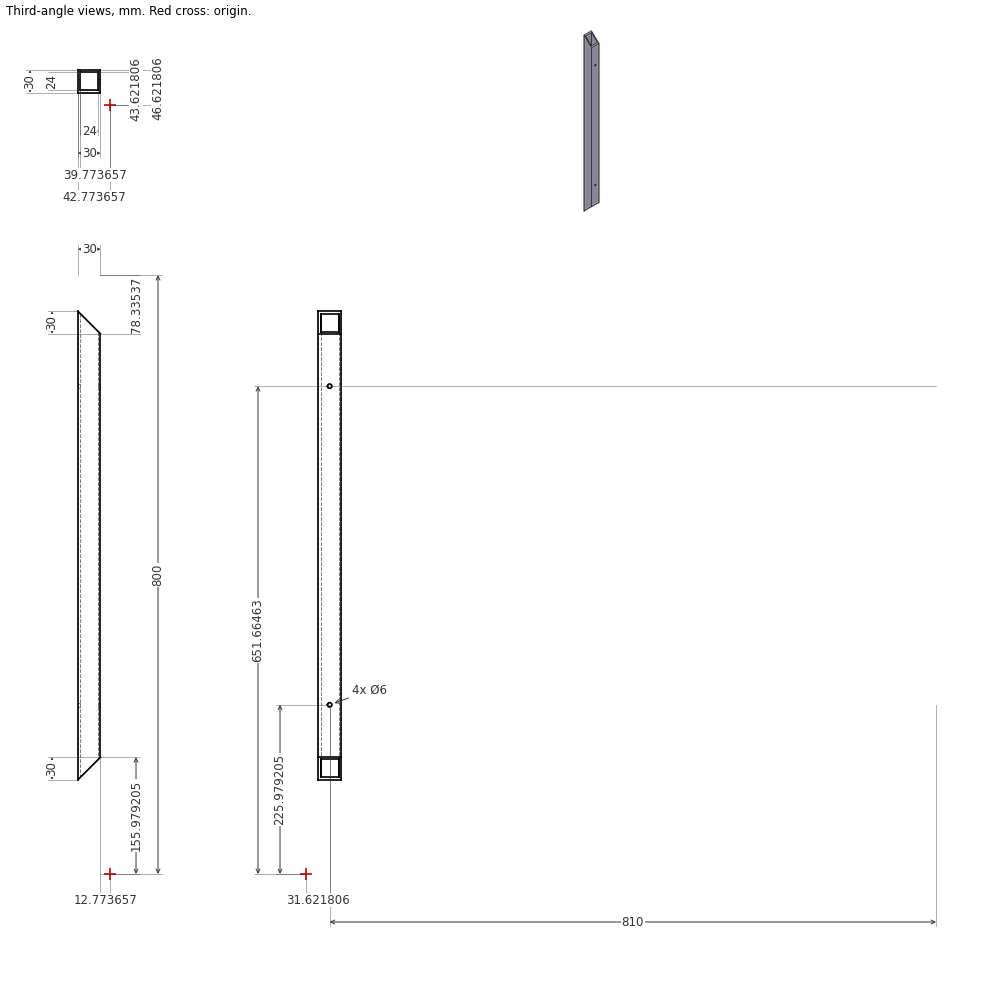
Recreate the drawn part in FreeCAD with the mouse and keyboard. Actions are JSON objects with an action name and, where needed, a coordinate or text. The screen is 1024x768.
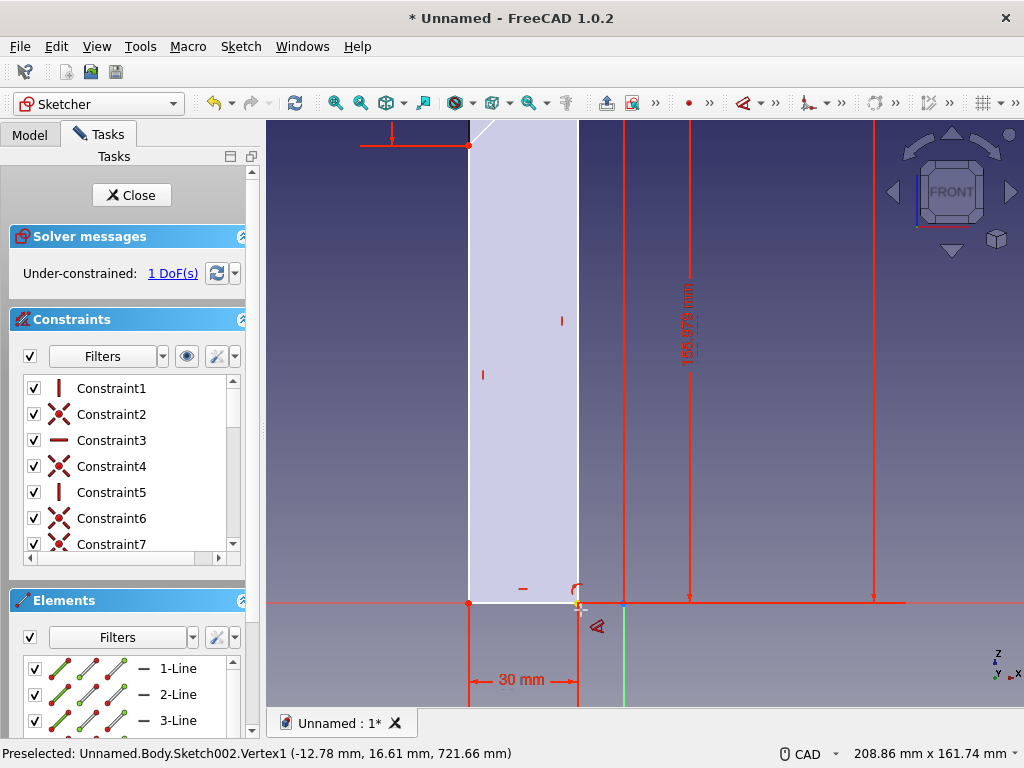
{"action": "left_click", "coordinate": [578, 603]}
{"action": "left_click", "coordinate": [601, 637]}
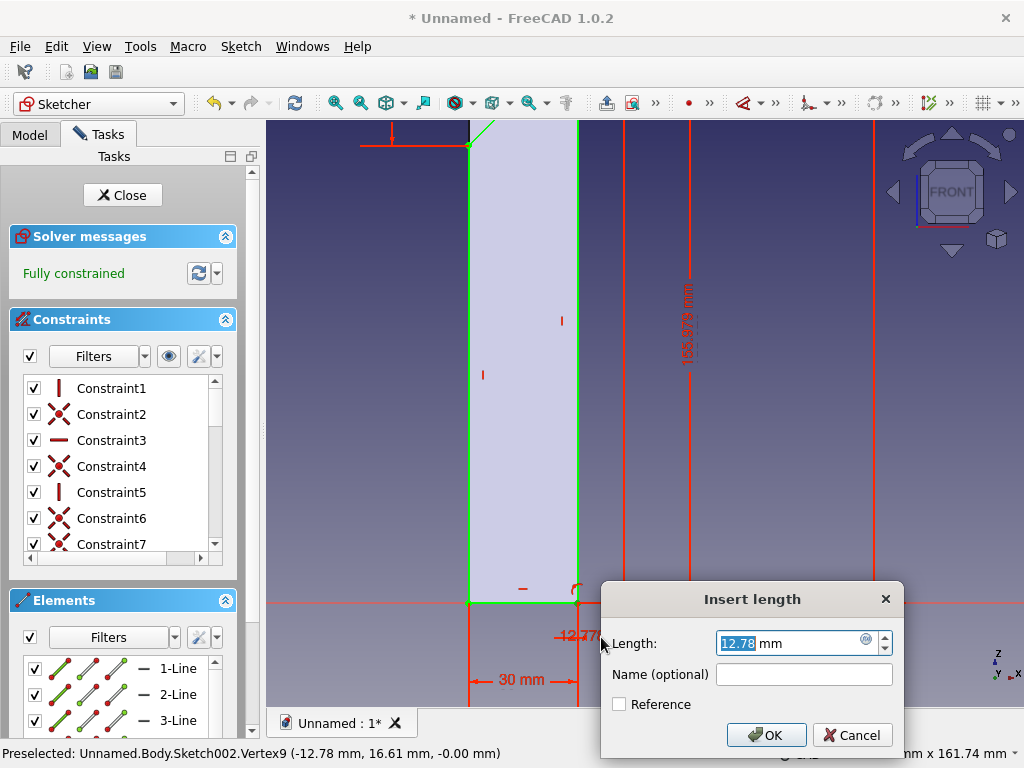
{"action": "type", "text": "12.773657"}
{"action": "key", "text": "Return"}
{"action": "key", "text": "Escape"}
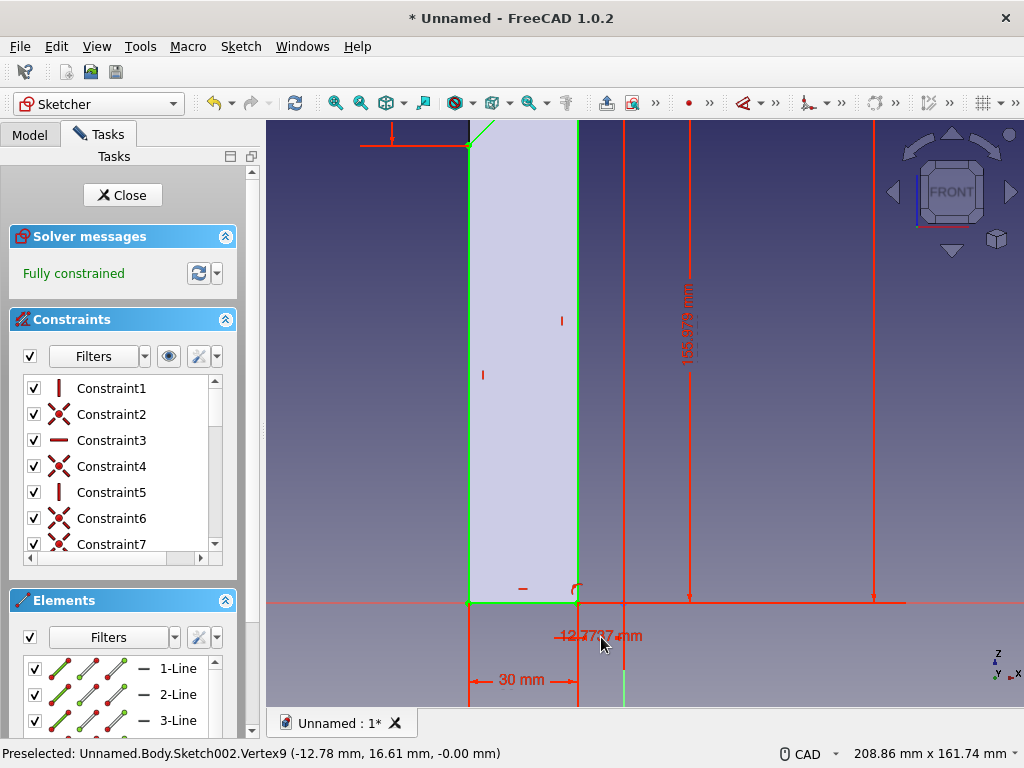
{"action": "left_click", "coordinate": [123, 195]}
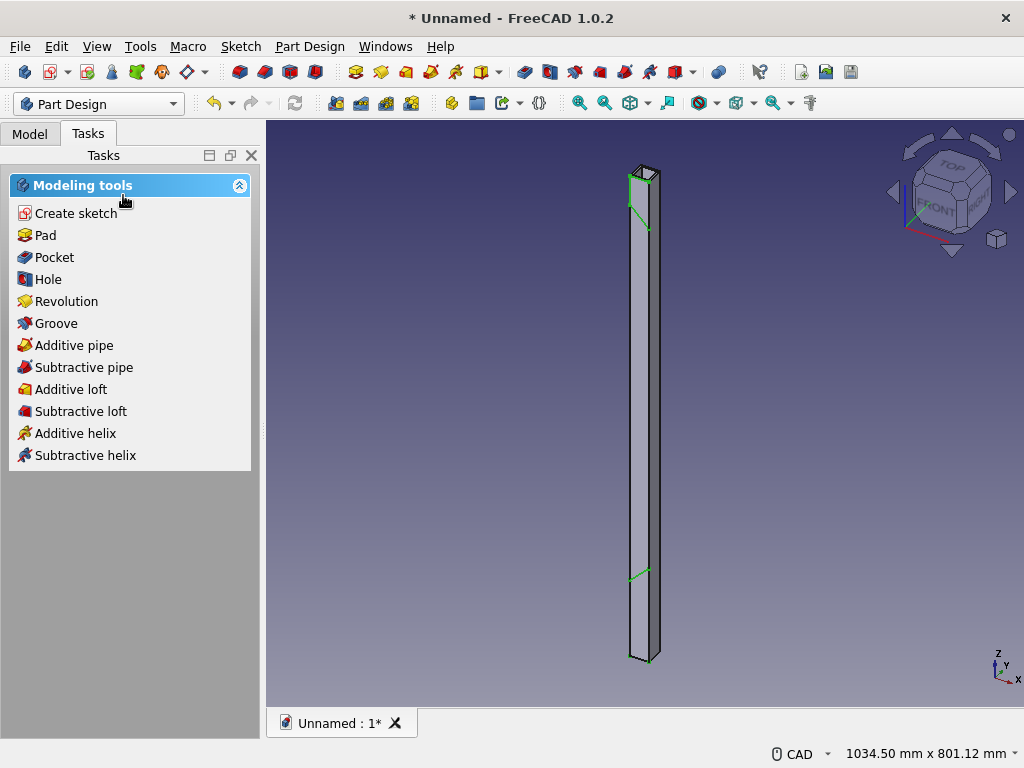
{"action": "left_click", "coordinate": [525, 72]}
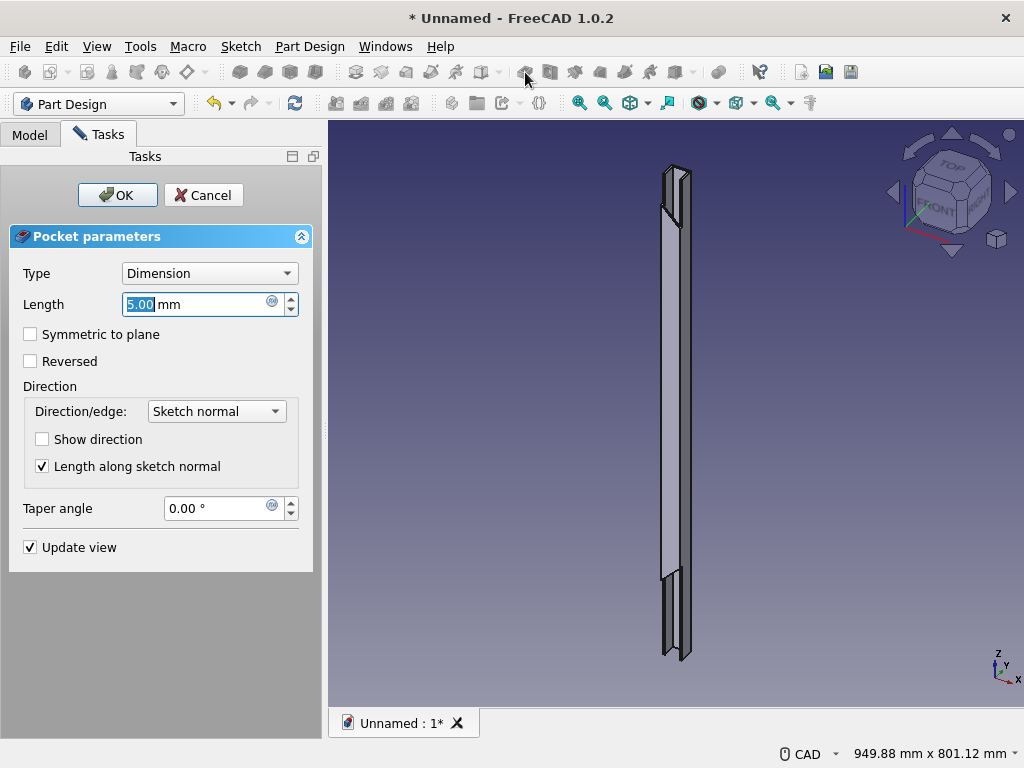
{"action": "left_click", "coordinate": [210, 274]}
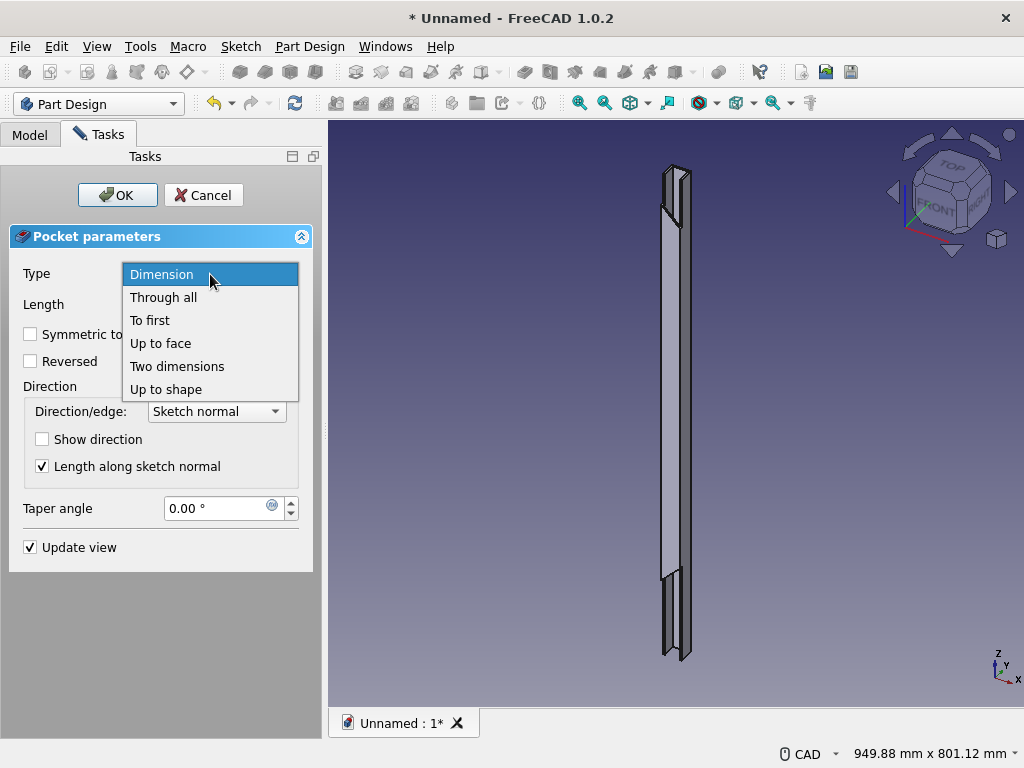
{"action": "left_click", "coordinate": [208, 298]}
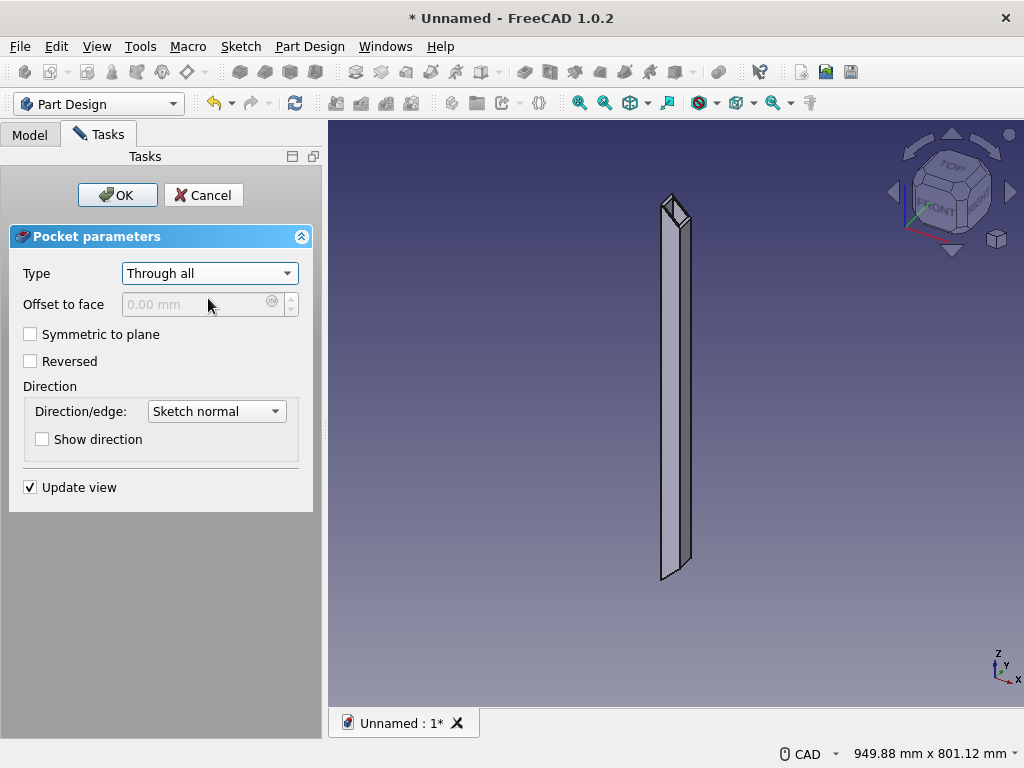
{"action": "left_click", "coordinate": [118, 195]}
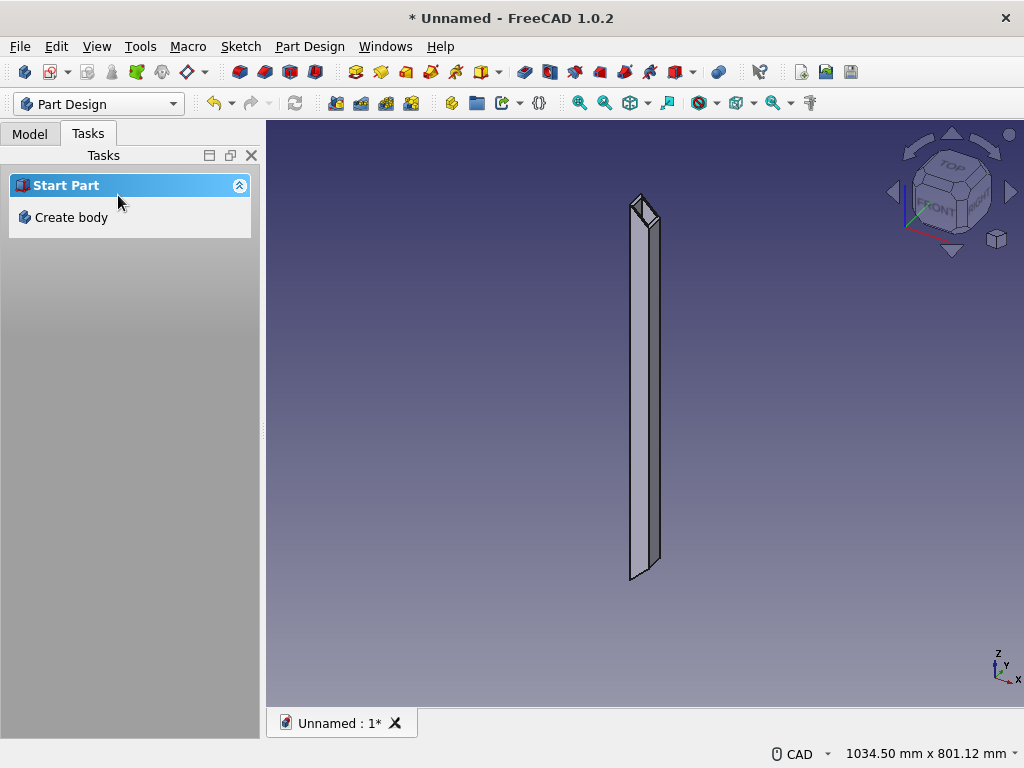
{"action": "left_click", "coordinate": [30, 134]}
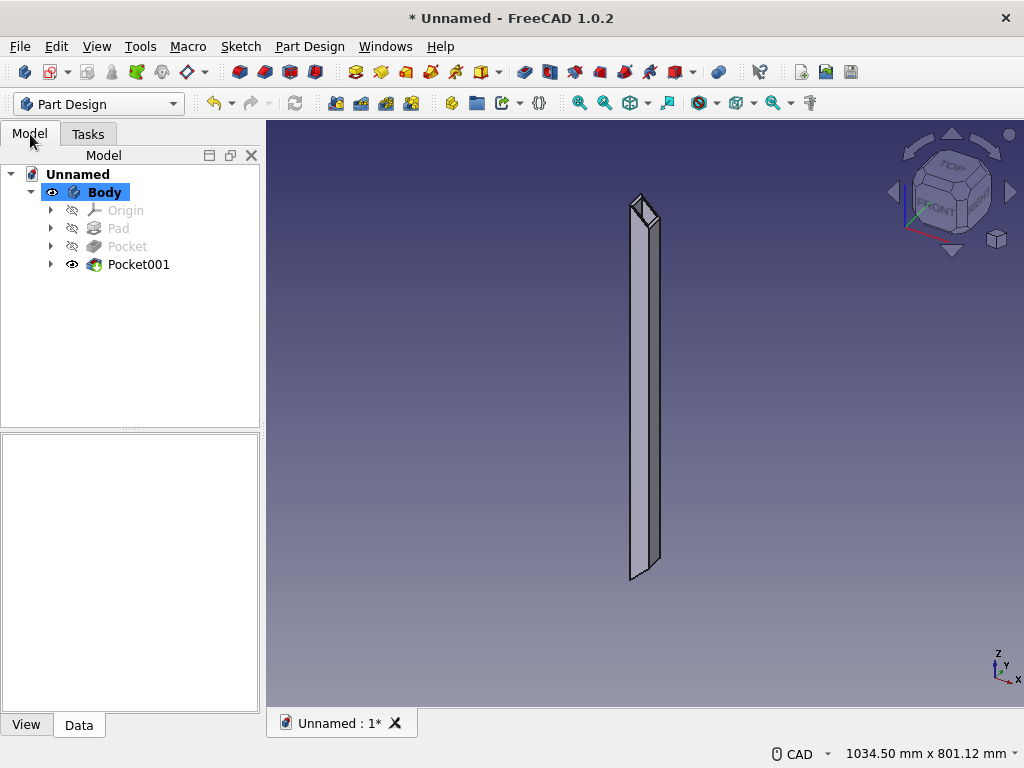
{"action": "left_click", "coordinate": [51, 210]}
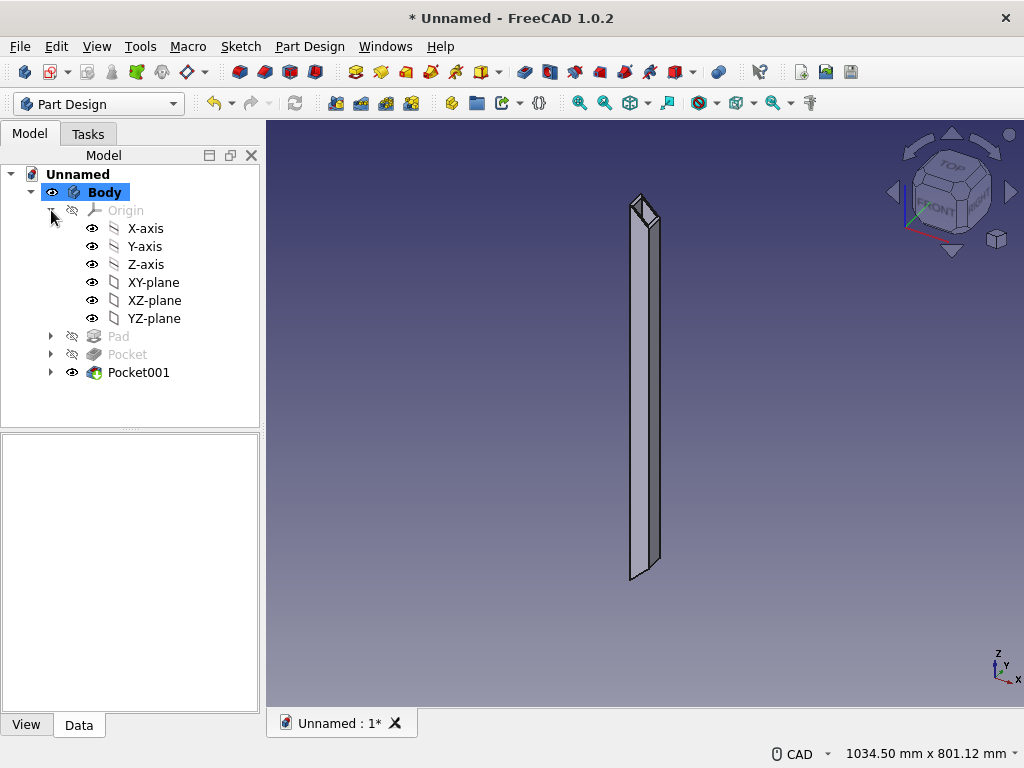
{"action": "left_click", "coordinate": [137, 318]}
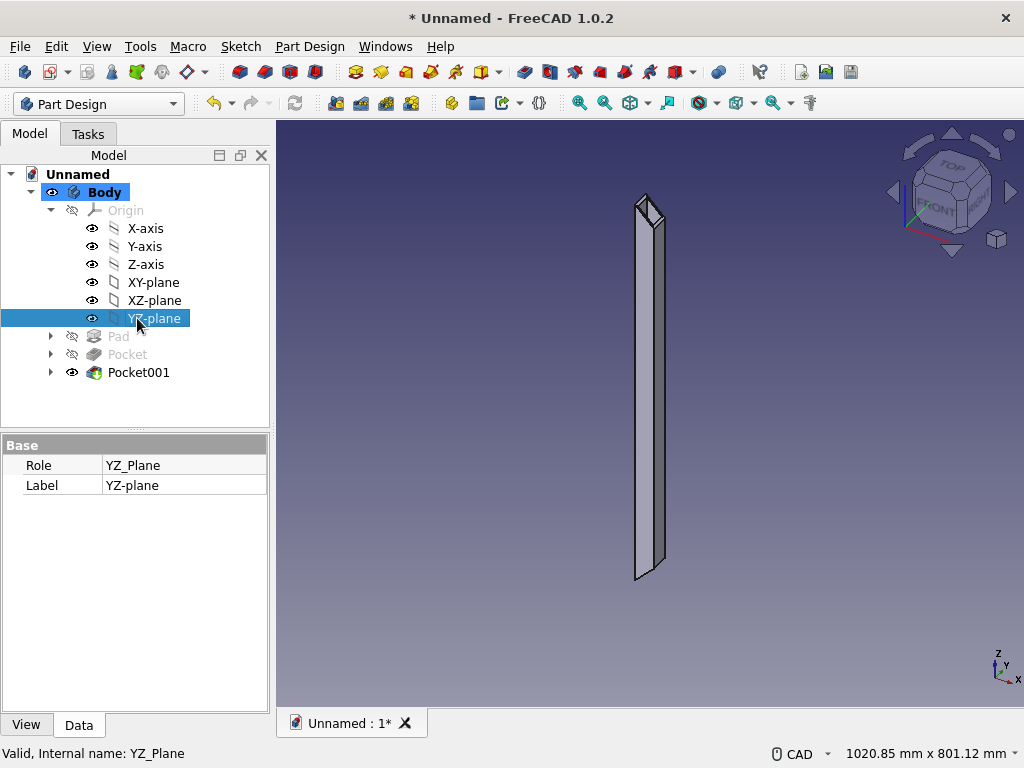
{"action": "left_click", "coordinate": [186, 72]}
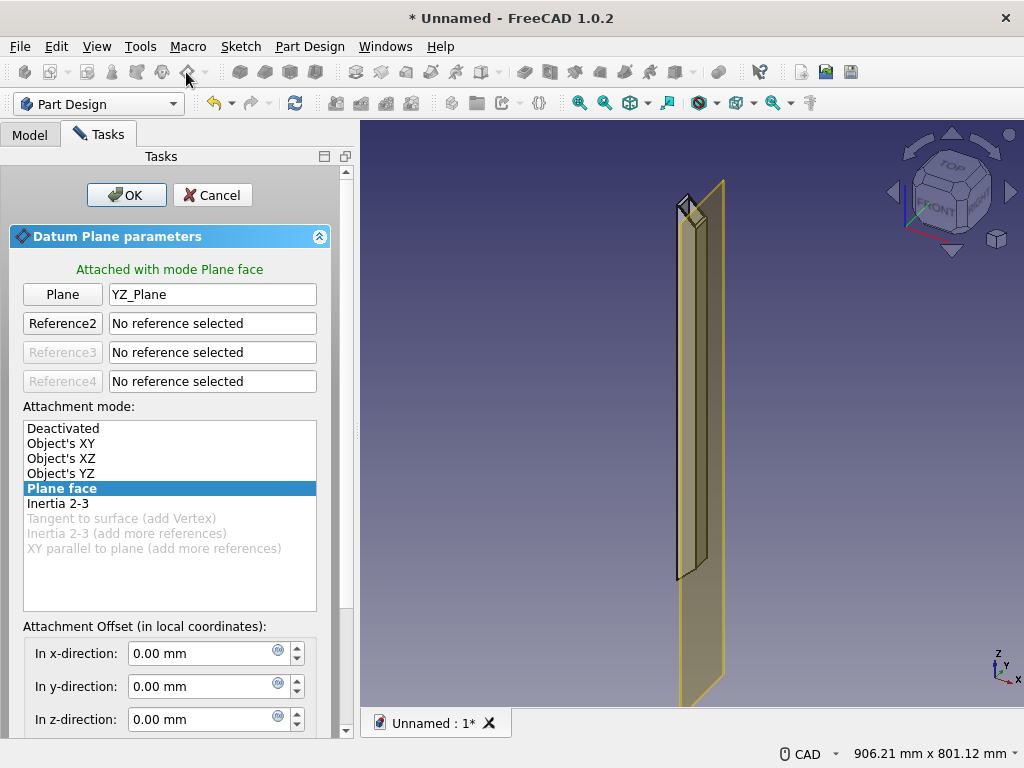
{"action": "triple_click", "coordinate": [210, 720]}